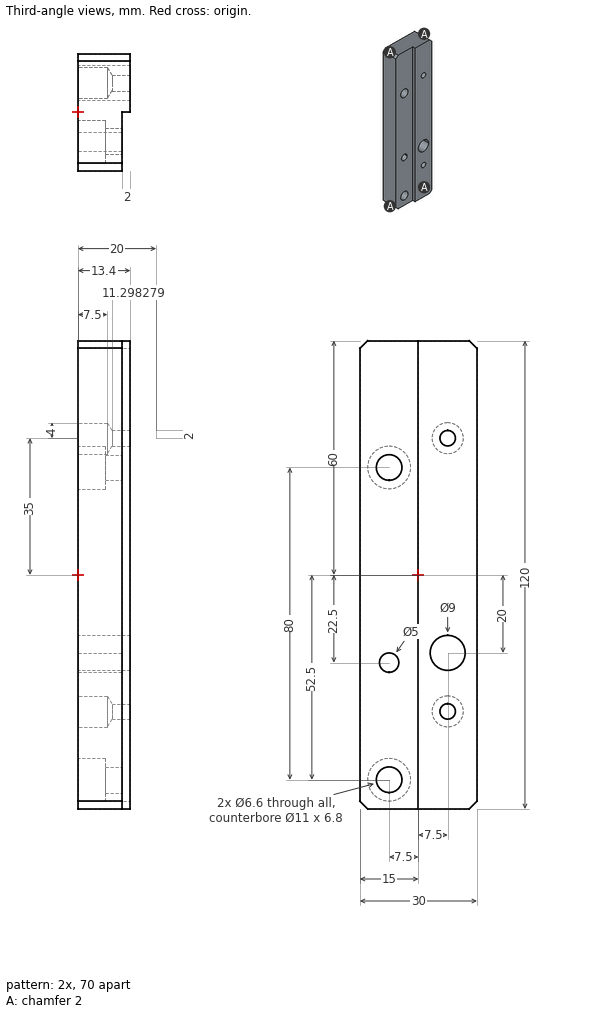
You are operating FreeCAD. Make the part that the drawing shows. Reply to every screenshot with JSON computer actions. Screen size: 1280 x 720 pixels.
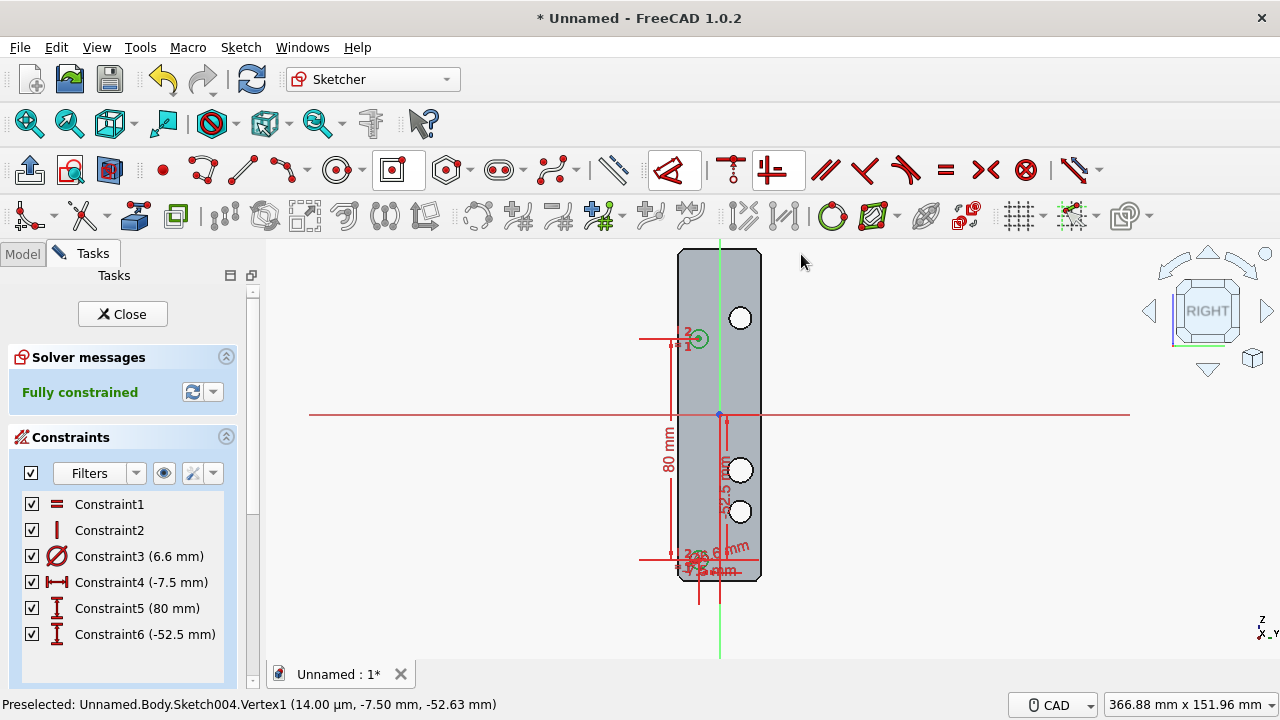
{"action": "left_click", "coordinate": [123, 314]}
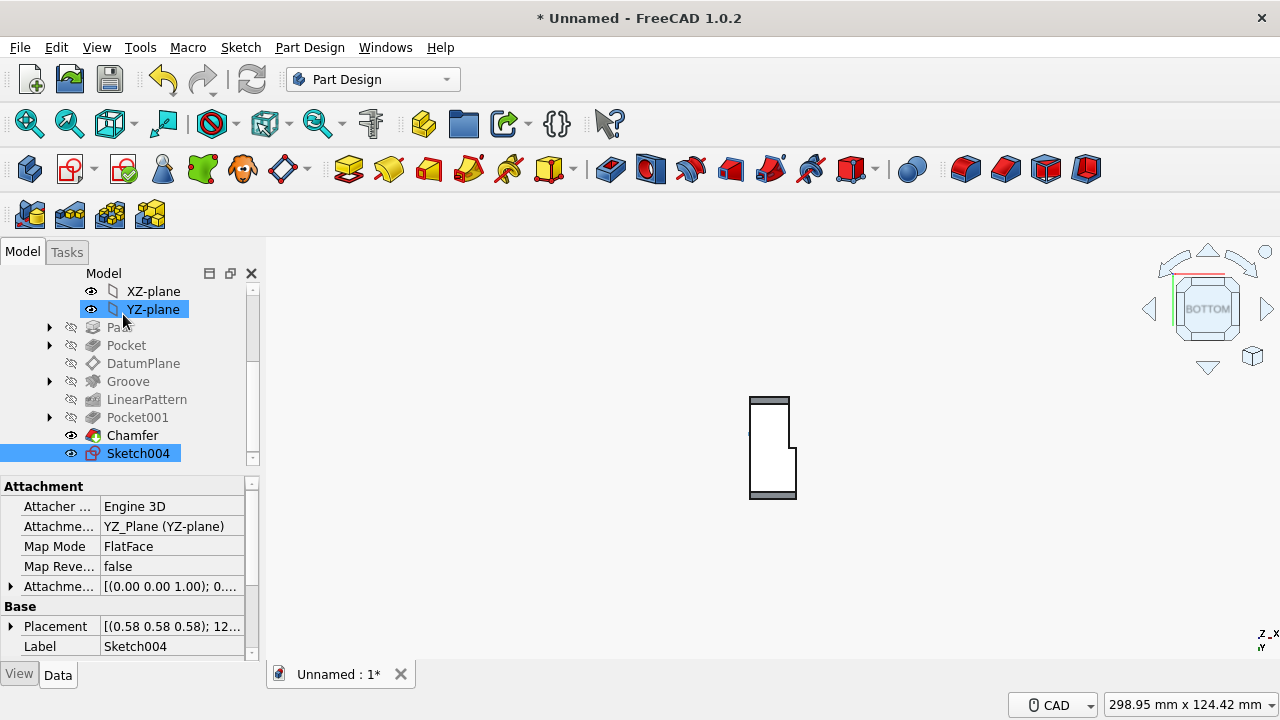
{"action": "left_click", "coordinate": [652, 170]}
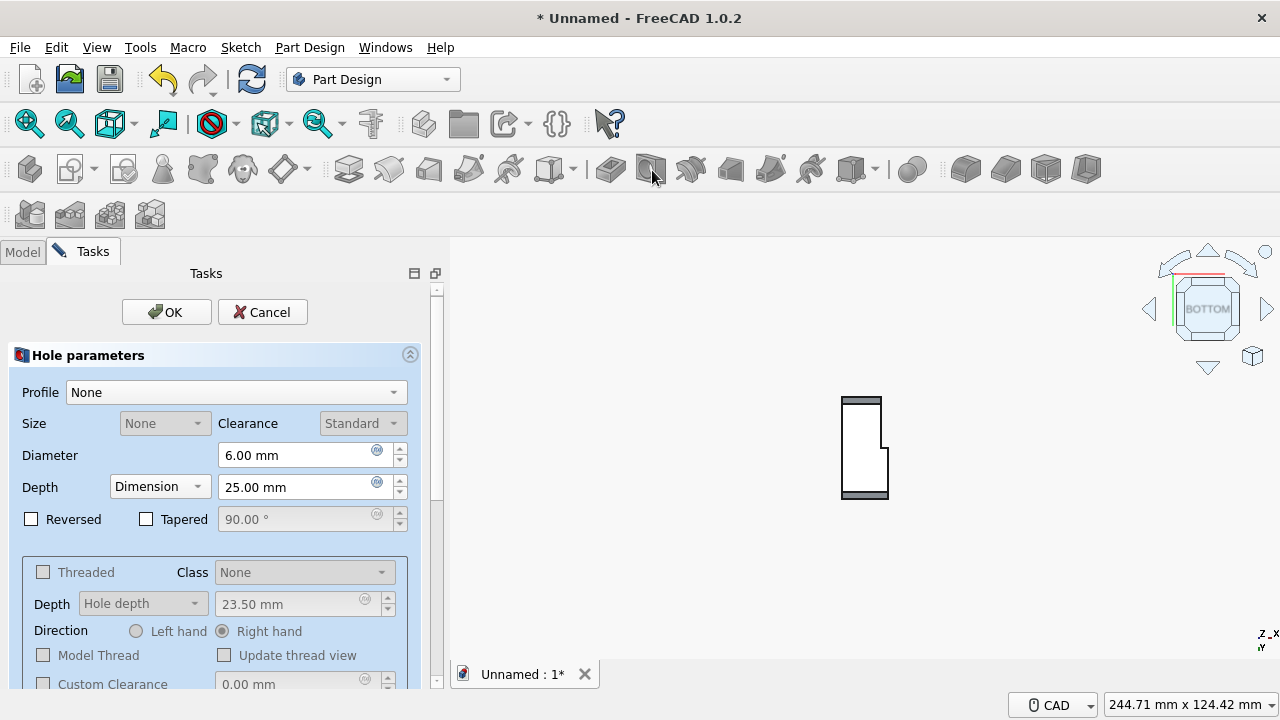
{"action": "triple_click", "coordinate": [305, 455]}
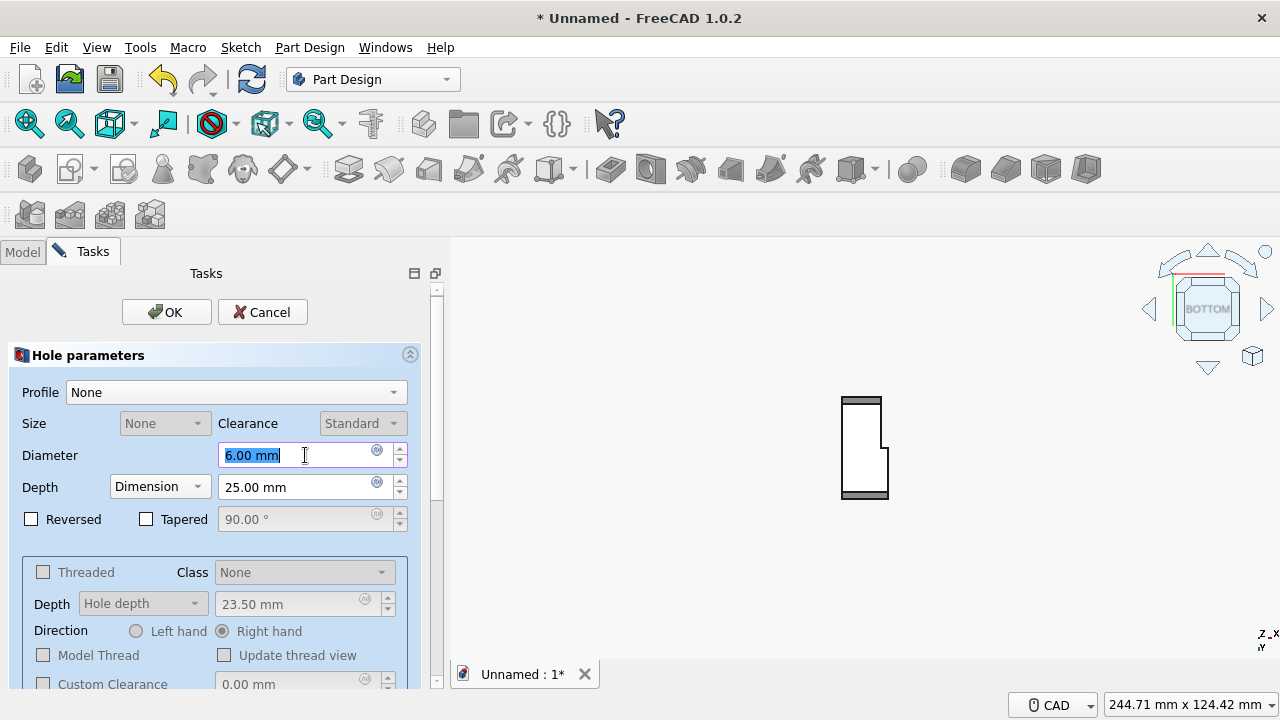
{"action": "type", "text": "6.6"}
{"action": "key", "text": "Tab"}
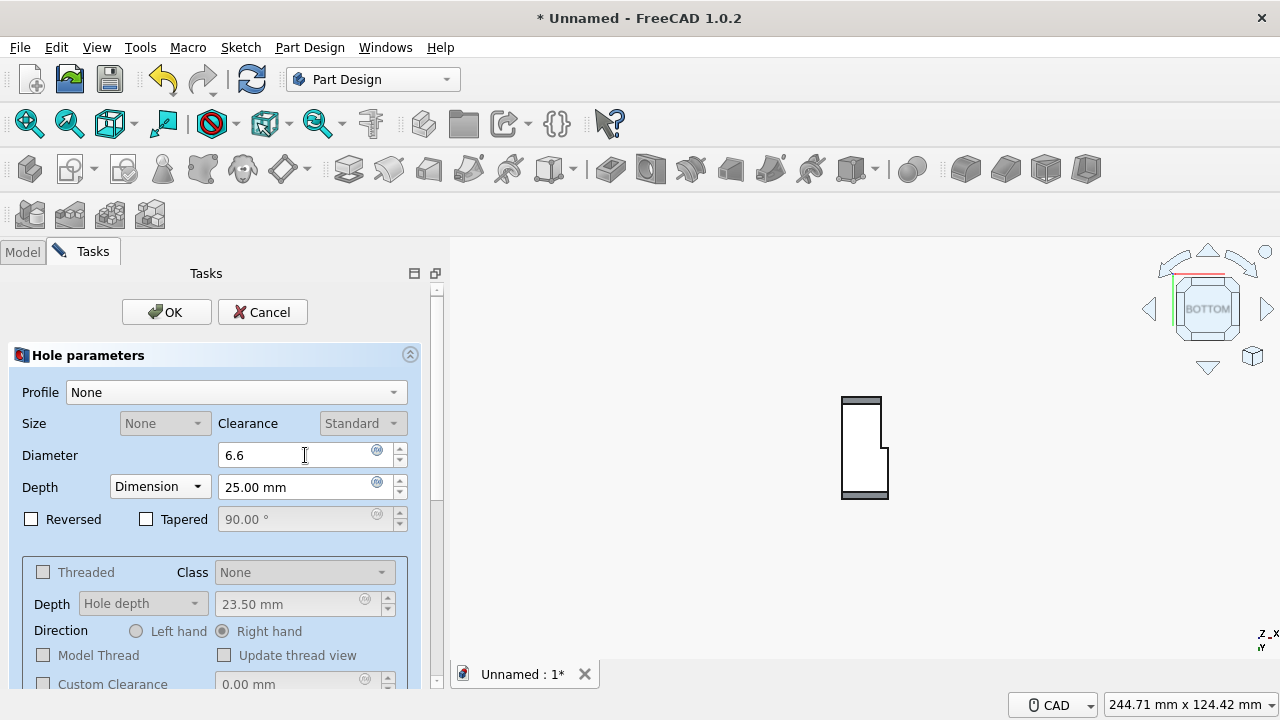
{"action": "left_click", "coordinate": [161, 486]}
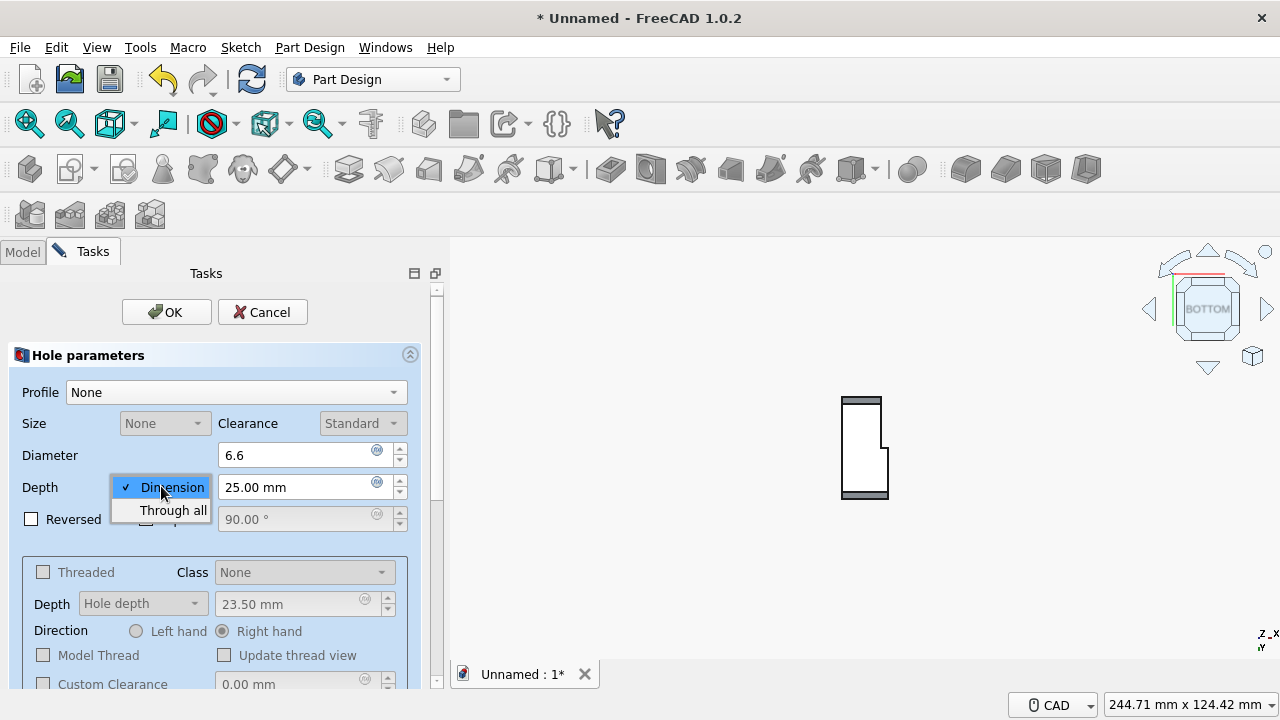
{"action": "left_click", "coordinate": [160, 510]}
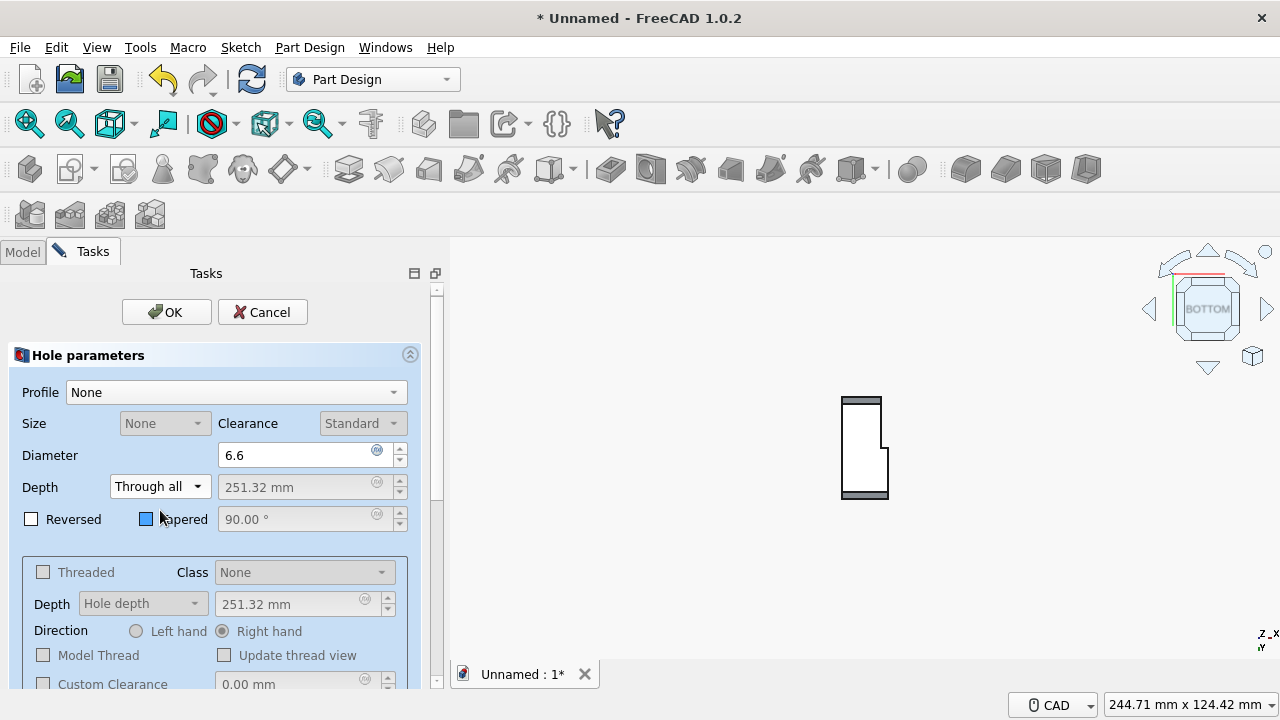
{"action": "left_click", "coordinate": [30, 519]}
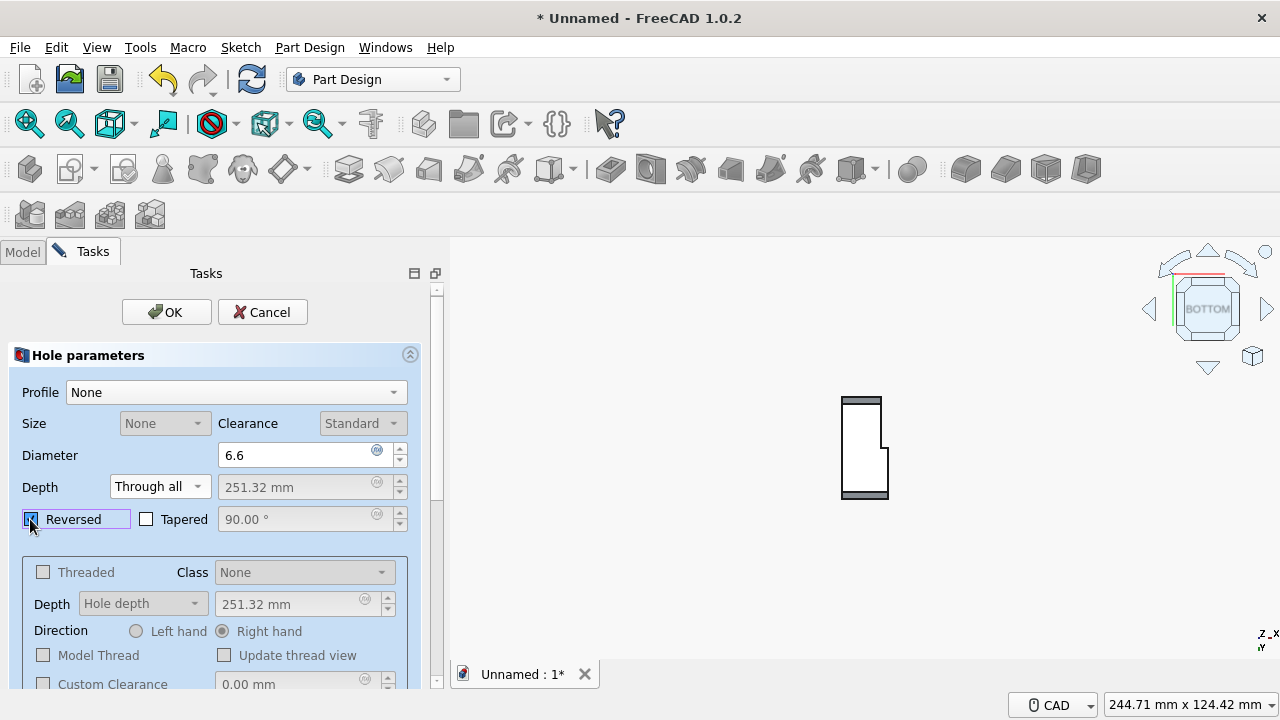
{"action": "scroll", "coordinate": [437, 486], "scroll_direction": "down", "scroll_amount": 3}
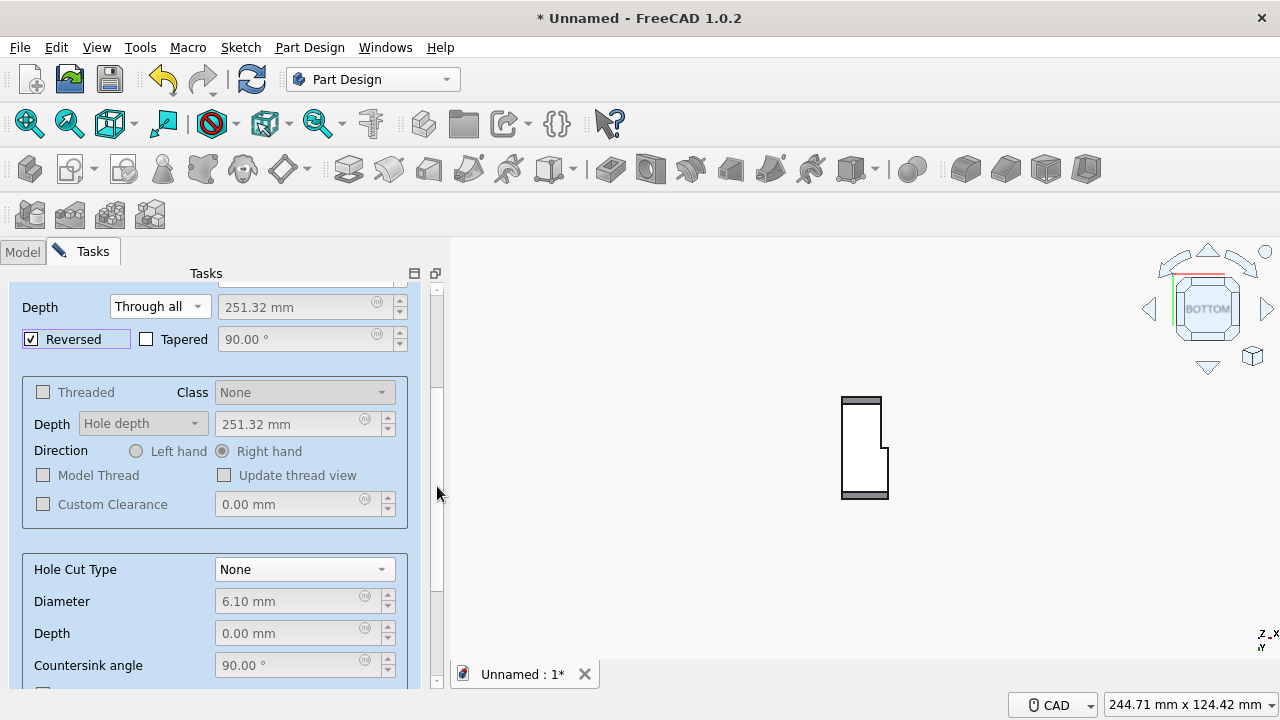
{"action": "left_click", "coordinate": [306, 570]}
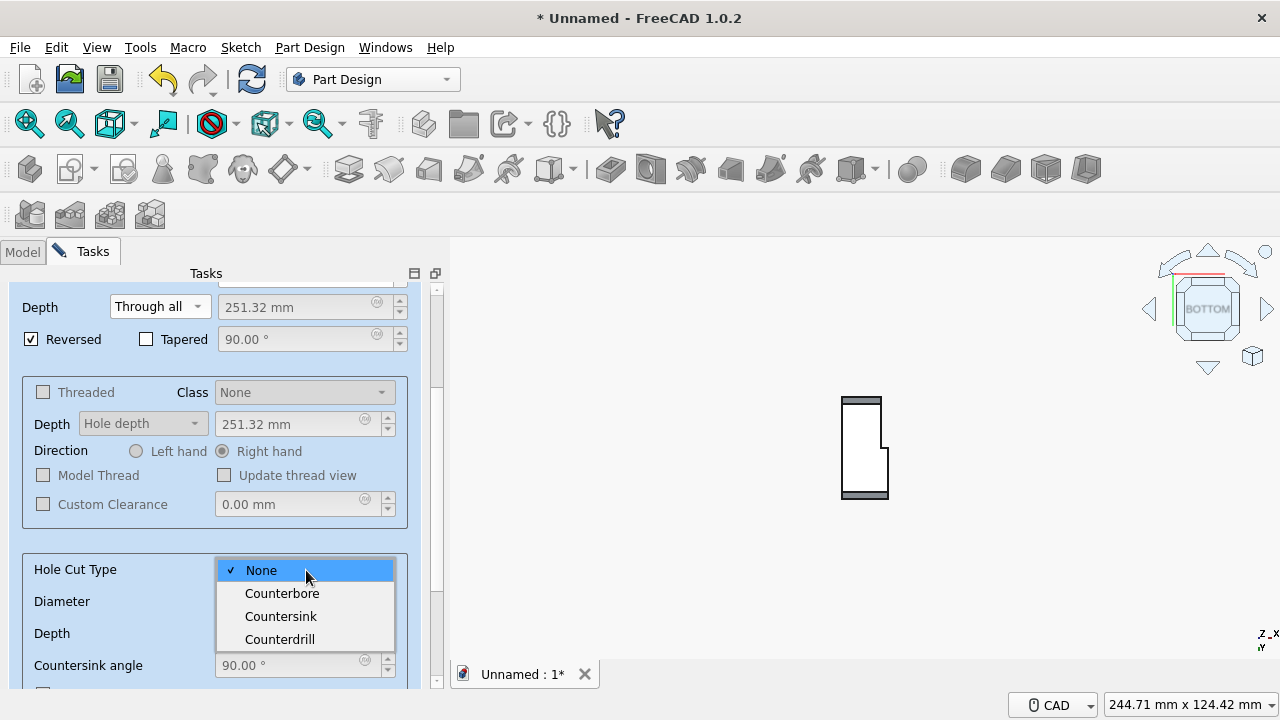
{"action": "left_click", "coordinate": [304, 594]}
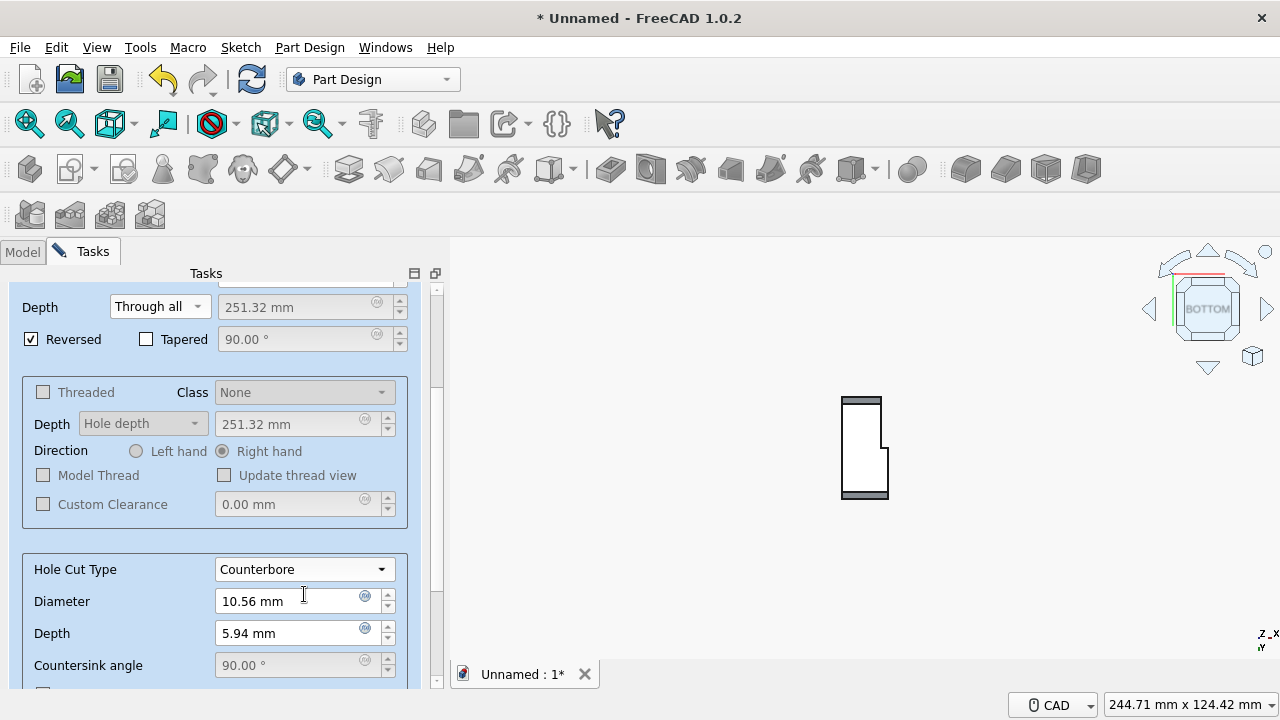
{"action": "triple_click", "coordinate": [298, 601]}